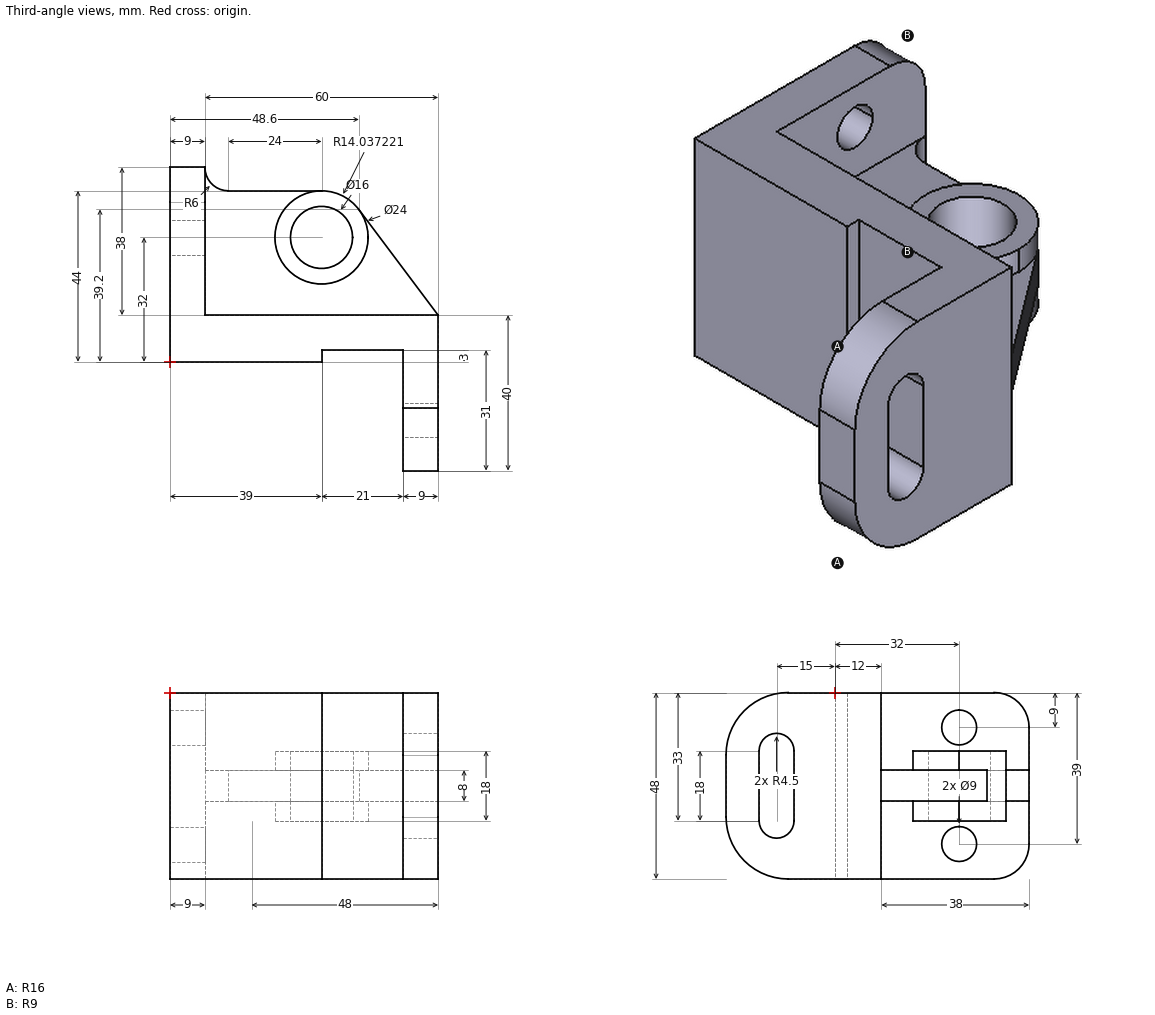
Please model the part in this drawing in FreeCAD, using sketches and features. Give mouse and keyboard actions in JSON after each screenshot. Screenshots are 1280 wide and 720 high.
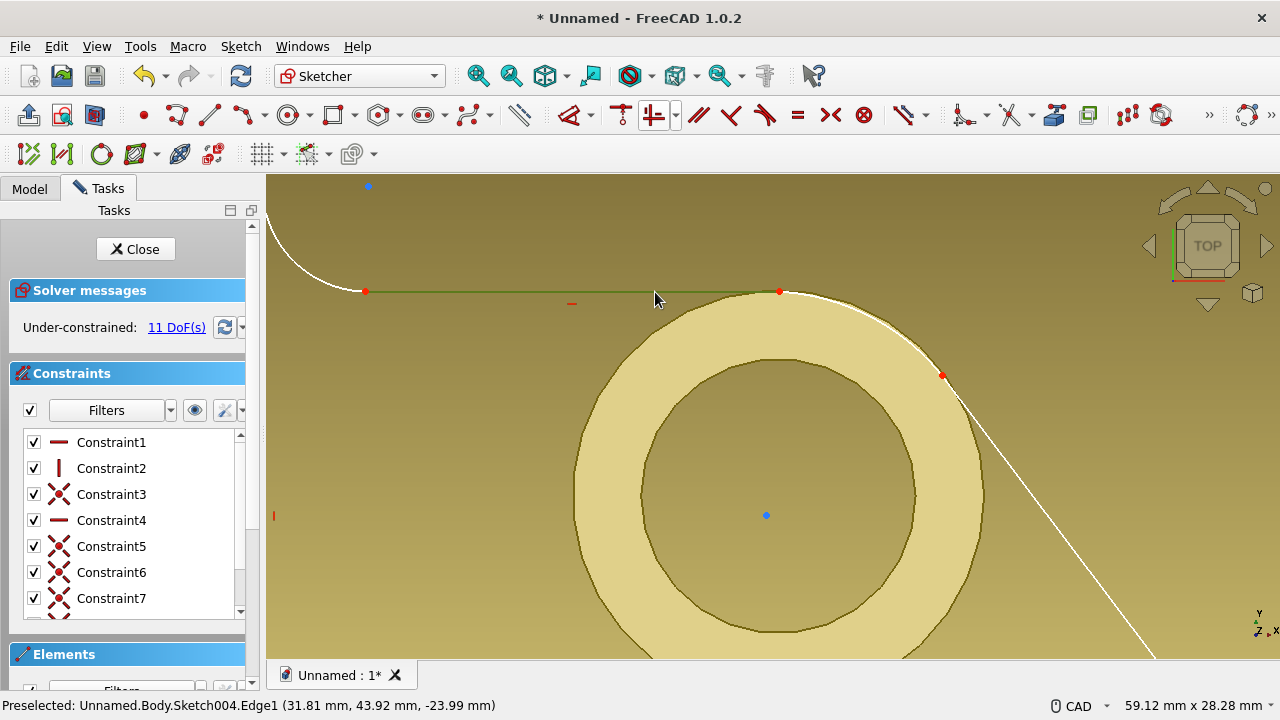
{"action": "left_click", "coordinate": [320, 280]}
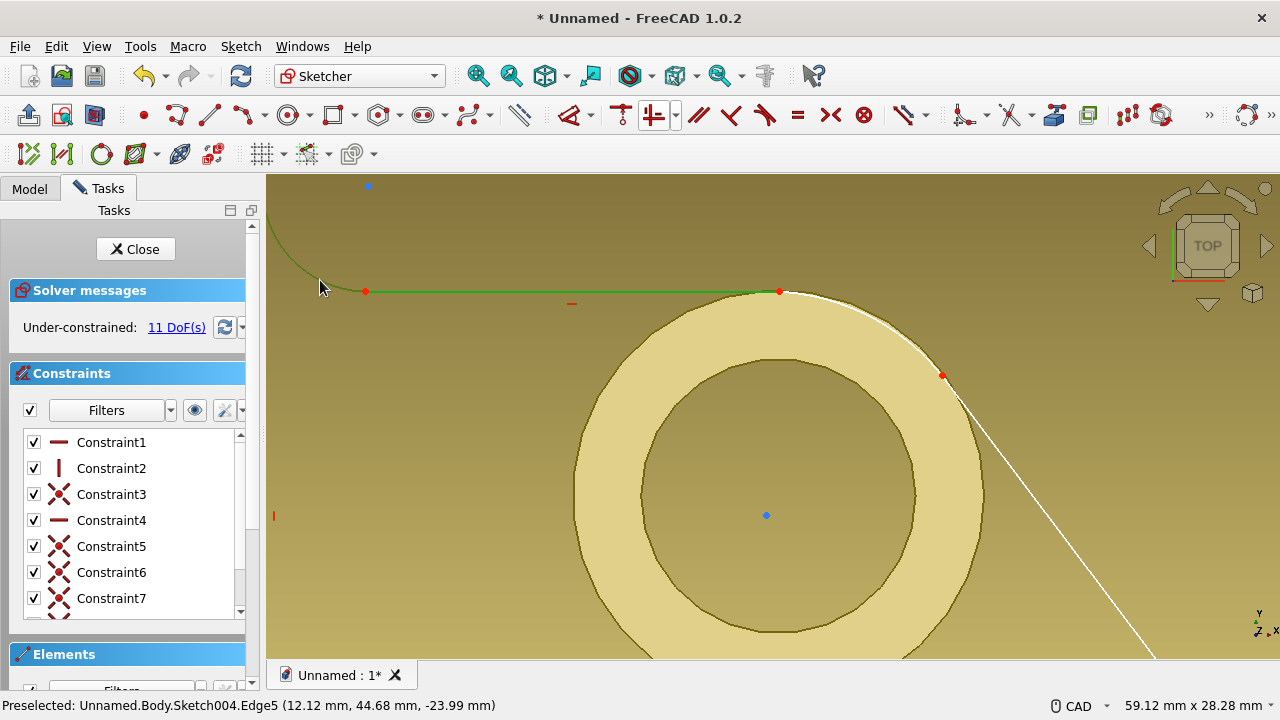
{"action": "left_click", "coordinate": [765, 116]}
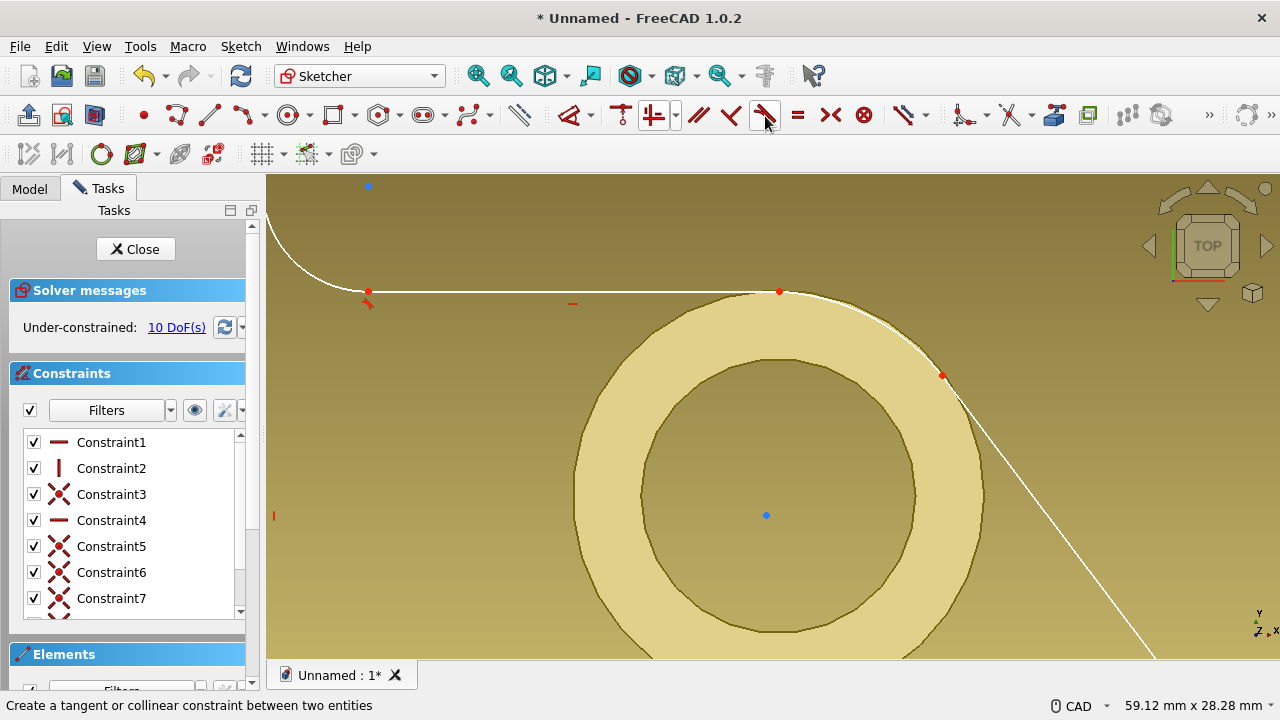
{"action": "scroll", "coordinate": [706, 300], "scroll_direction": "down", "scroll_amount": 5}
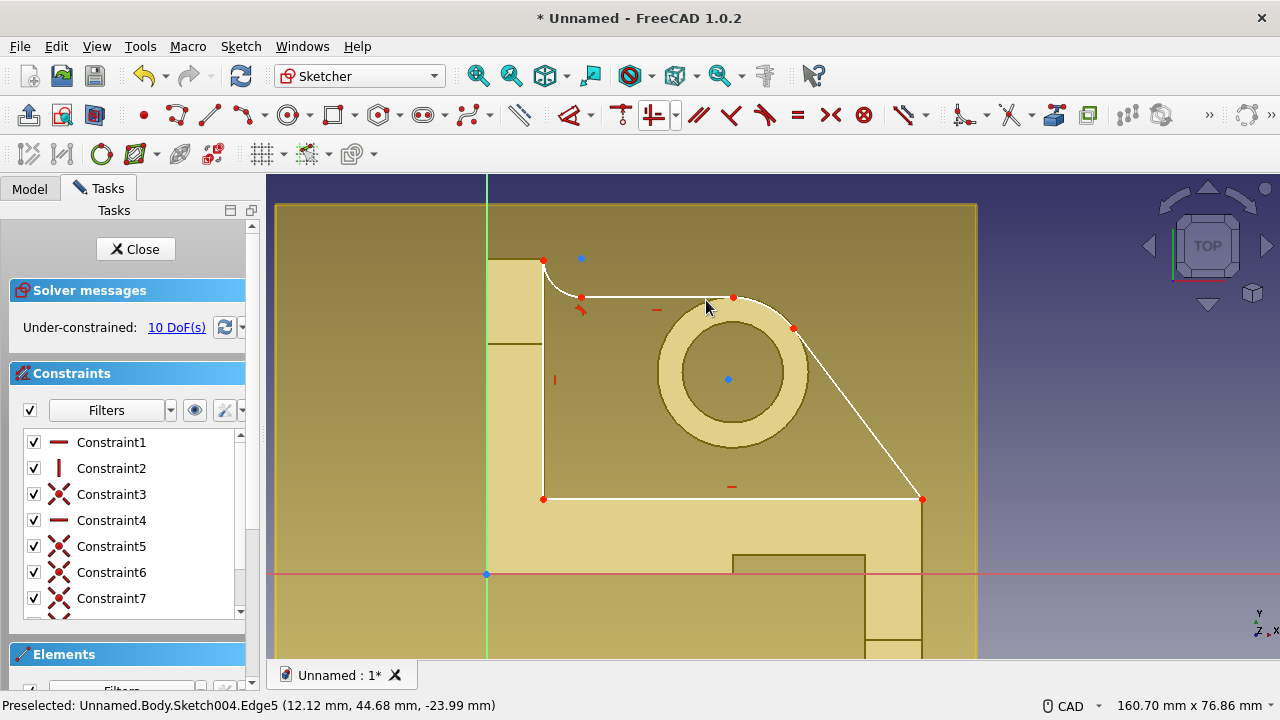
{"action": "left_click", "coordinate": [543, 332]}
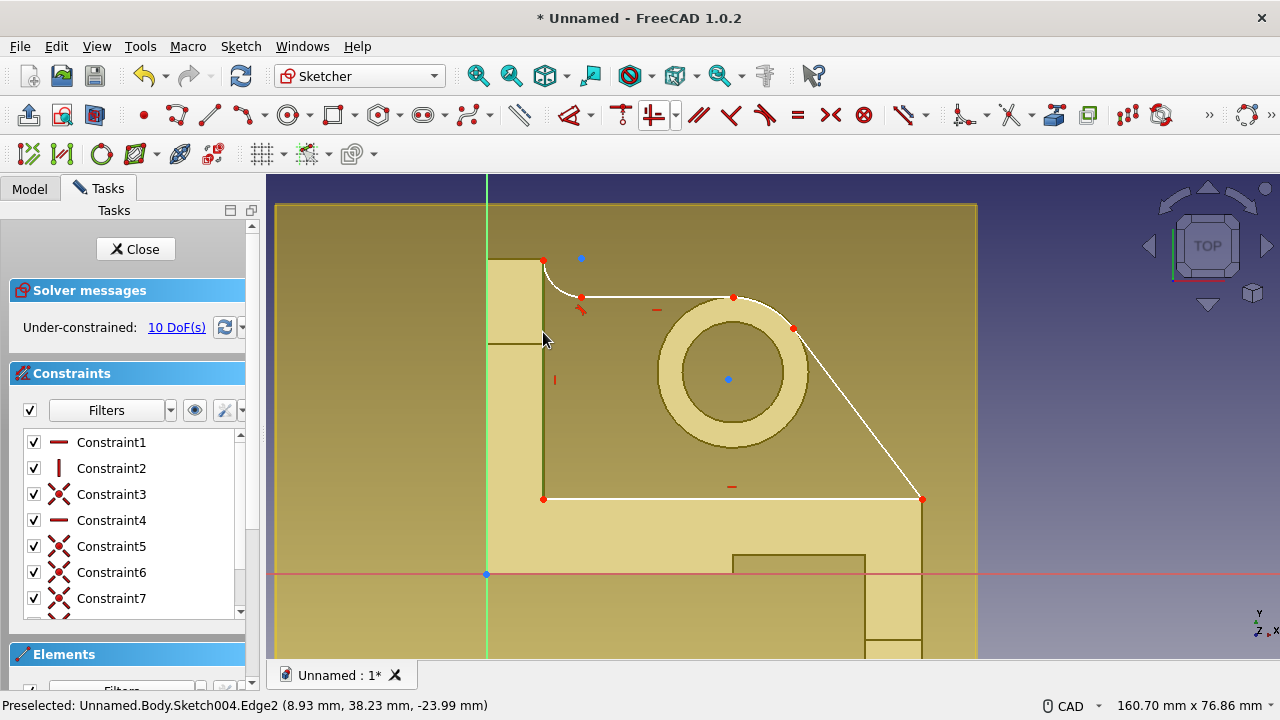
{"action": "left_click", "coordinate": [565, 293]}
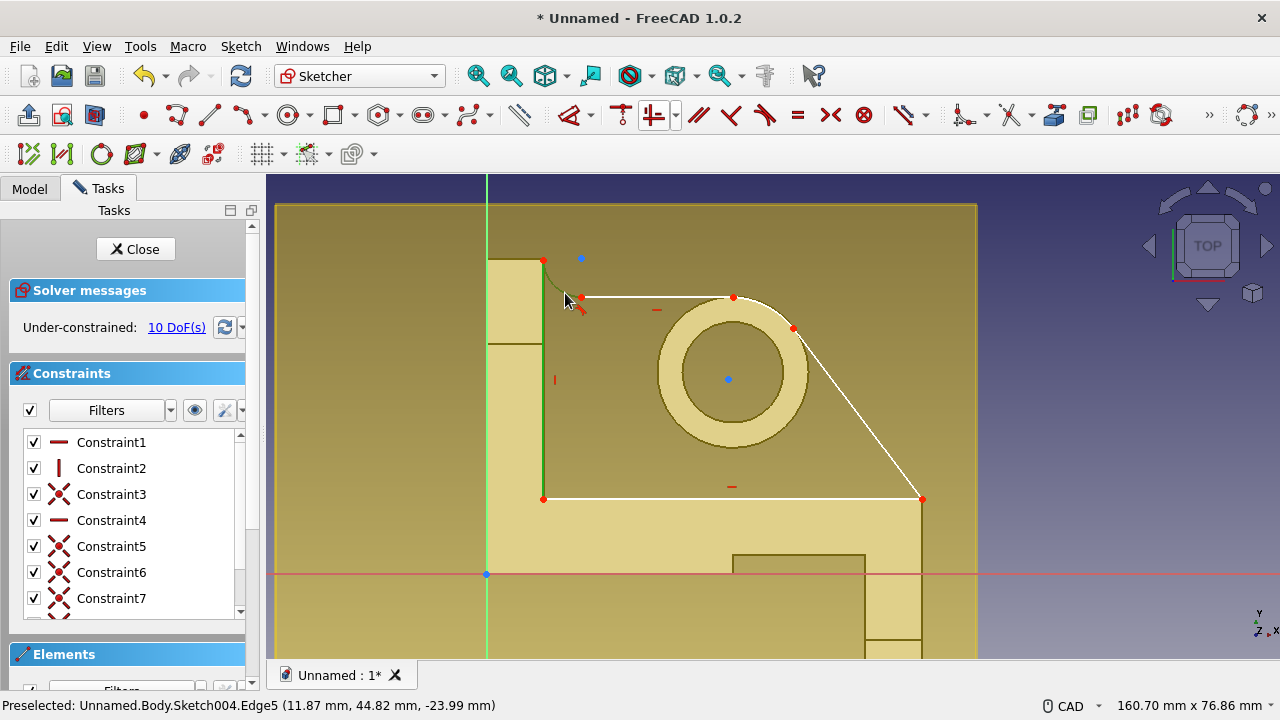
{"action": "key", "text": "t"}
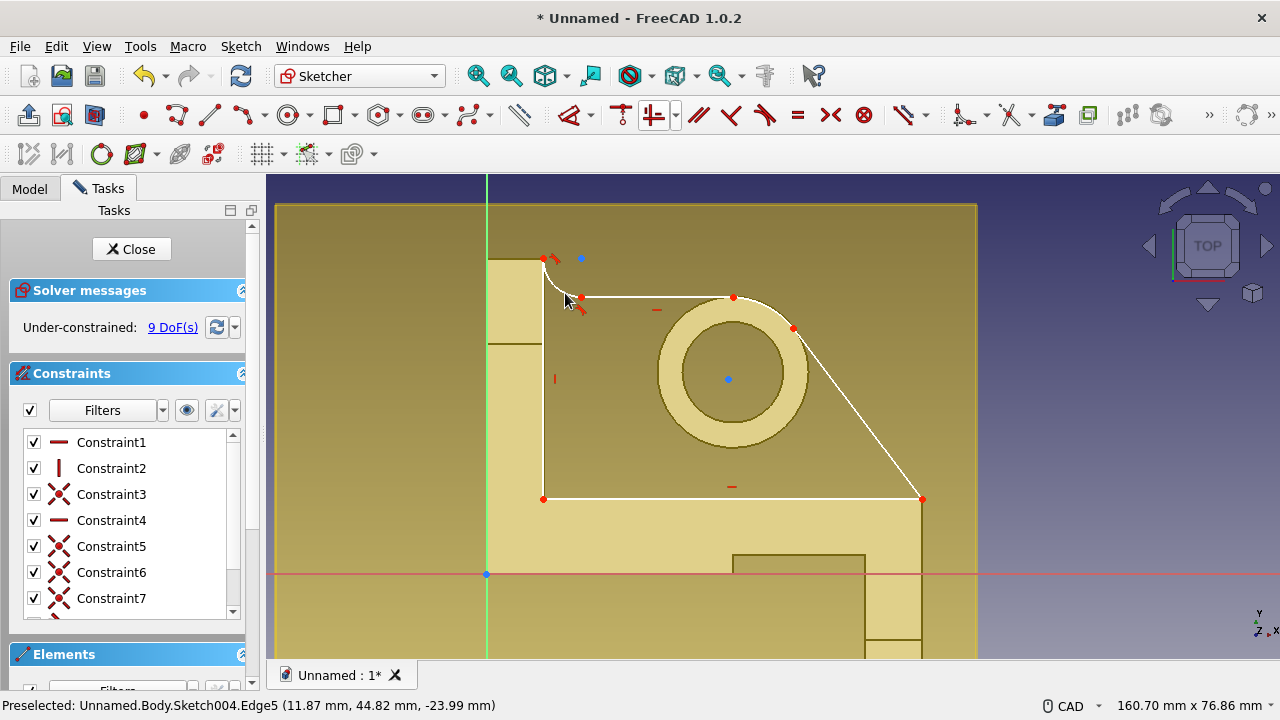
{"action": "key", "text": "d"}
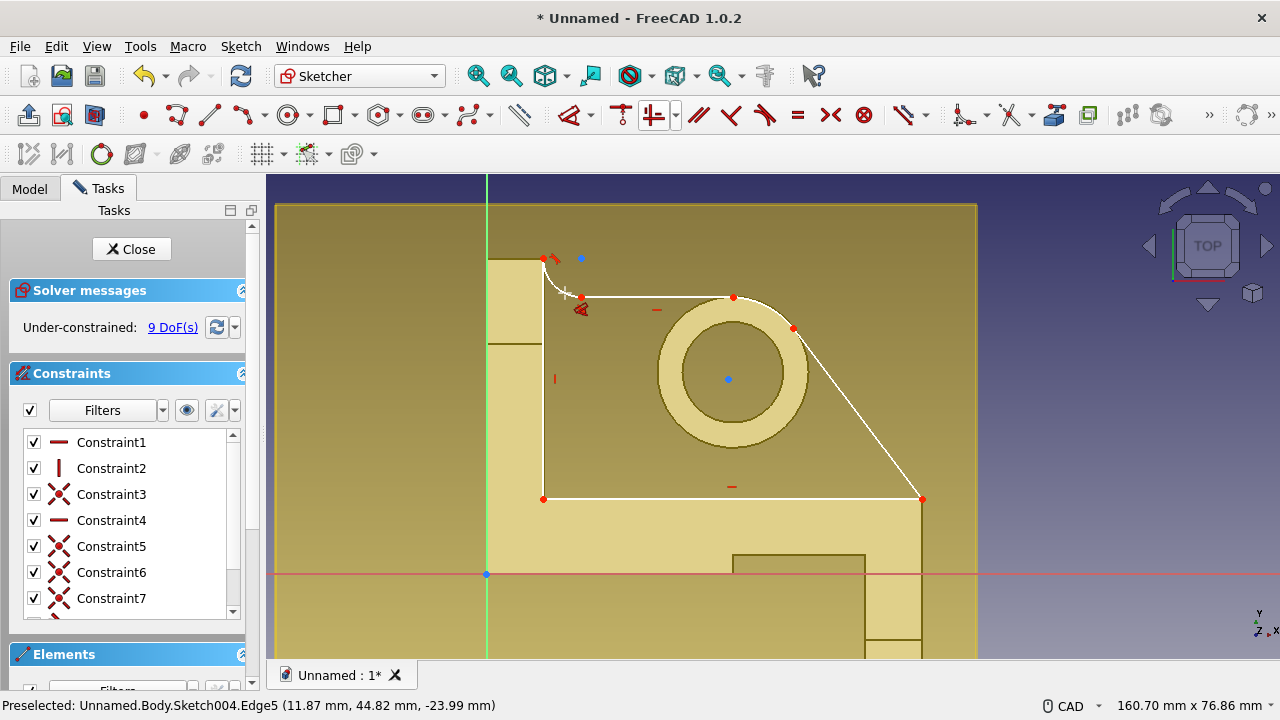
{"action": "left_click", "coordinate": [564, 293]}
{"action": "left_click", "coordinate": [523, 298]}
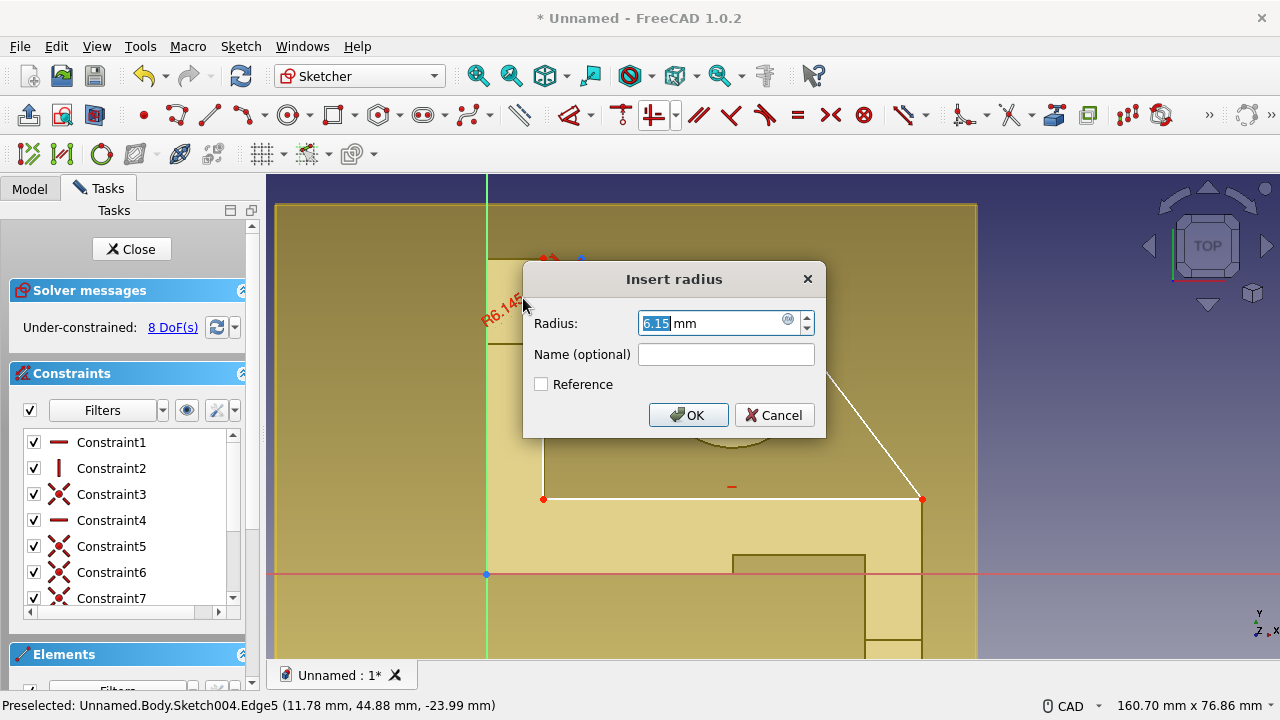
{"action": "type", "text": "6"}
{"action": "key", "text": "Return"}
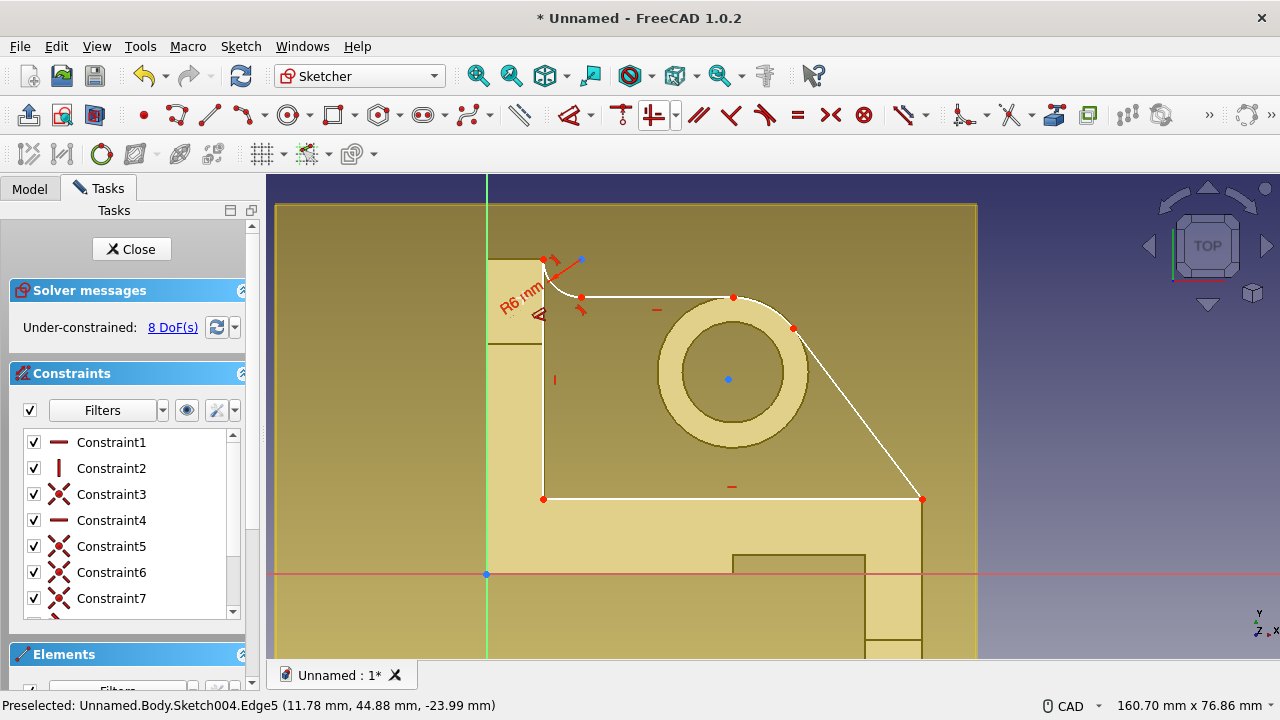
{"action": "left_click", "coordinate": [778, 314]}
{"action": "left_click", "coordinate": [797, 288]}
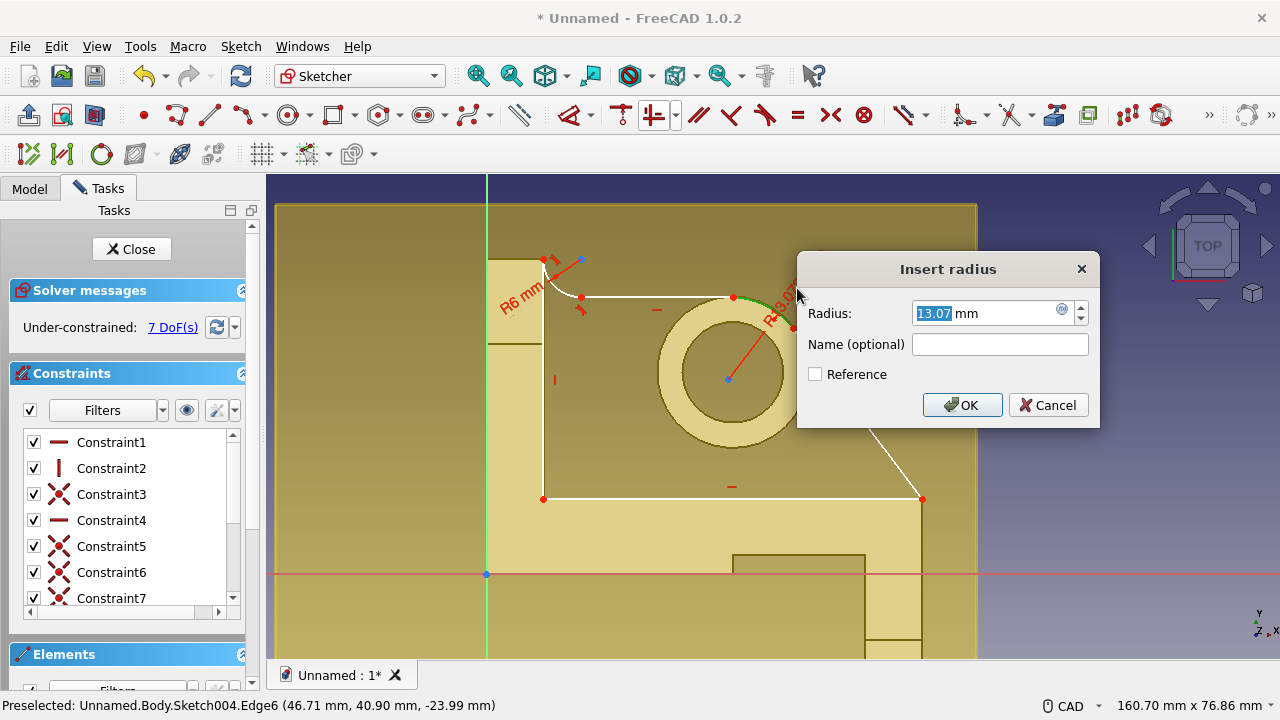
{"action": "type", "text": "14.037221"}
{"action": "key", "text": "Return"}